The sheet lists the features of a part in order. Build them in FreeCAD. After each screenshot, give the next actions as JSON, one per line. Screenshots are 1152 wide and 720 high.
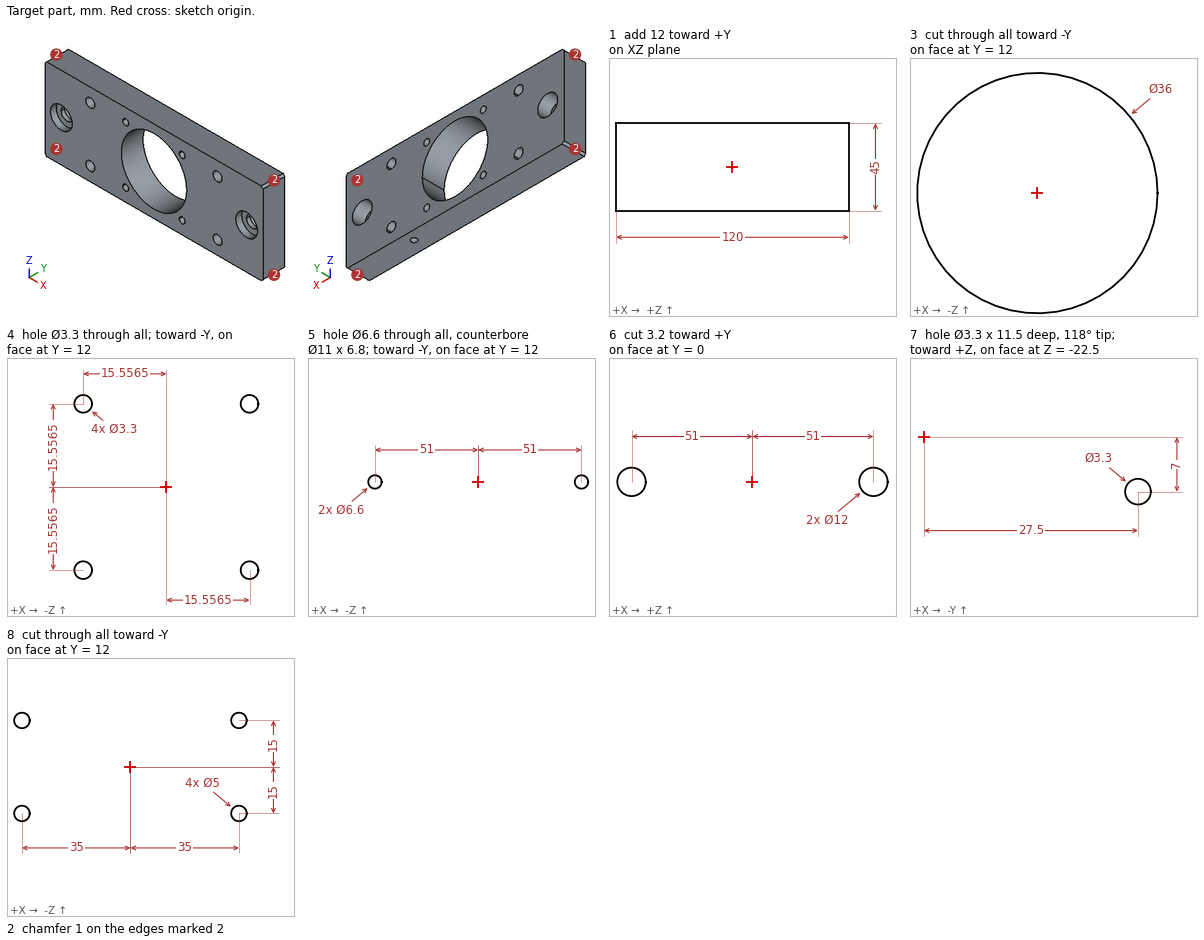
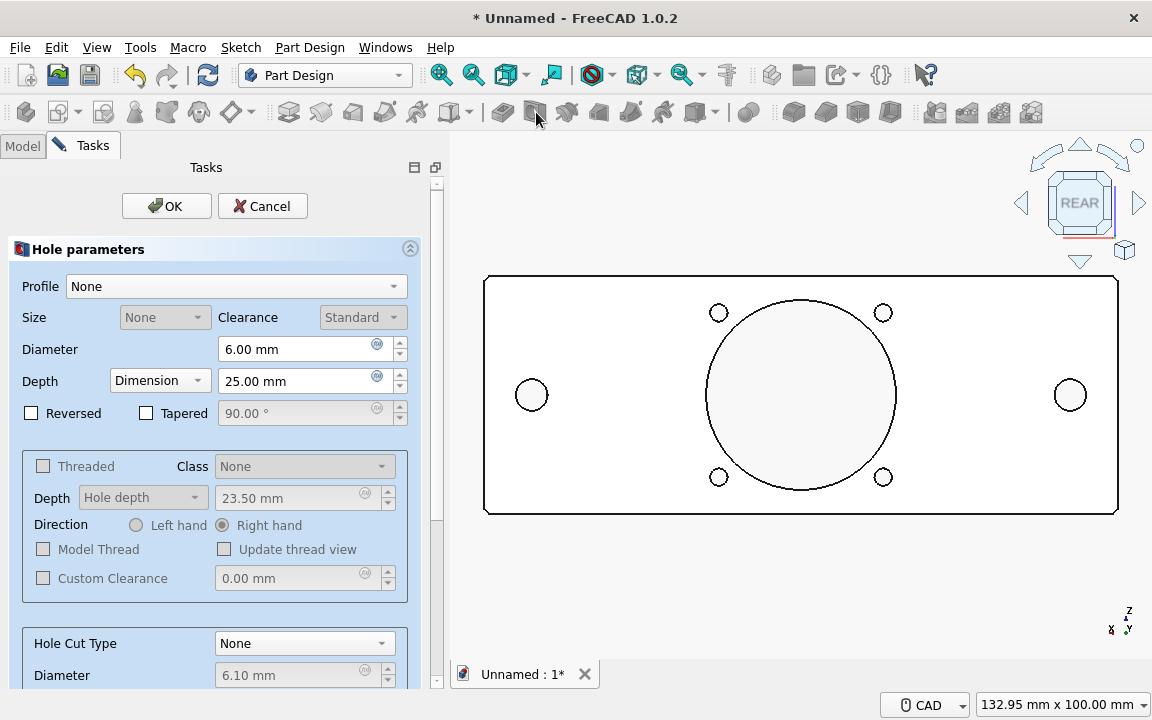
{"action": "triple_click", "coordinate": [305, 349]}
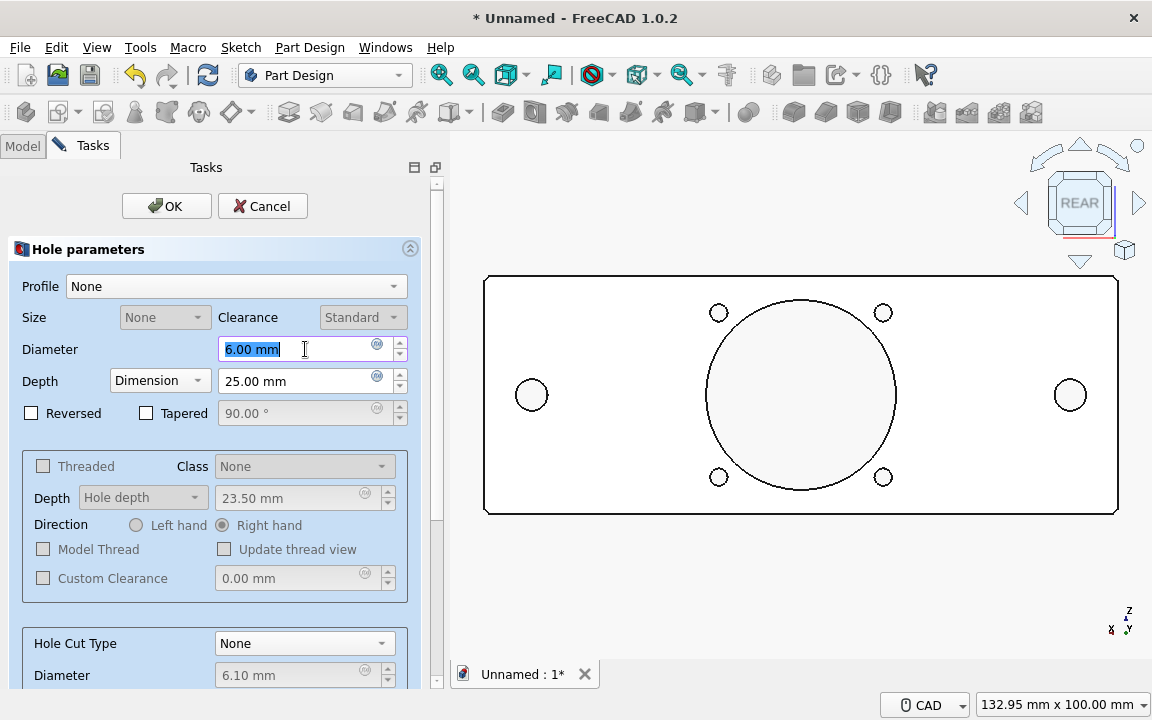
{"action": "type", "text": "6.6"}
{"action": "key", "text": "Tab"}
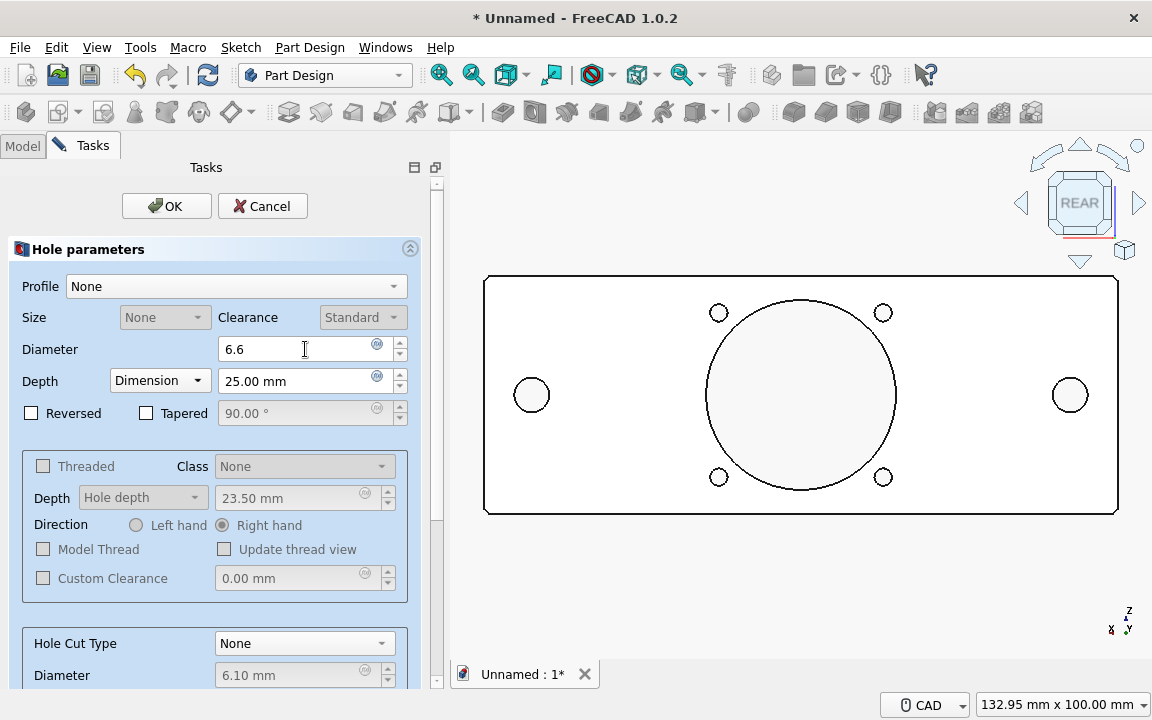
{"action": "left_click", "coordinate": [161, 380]}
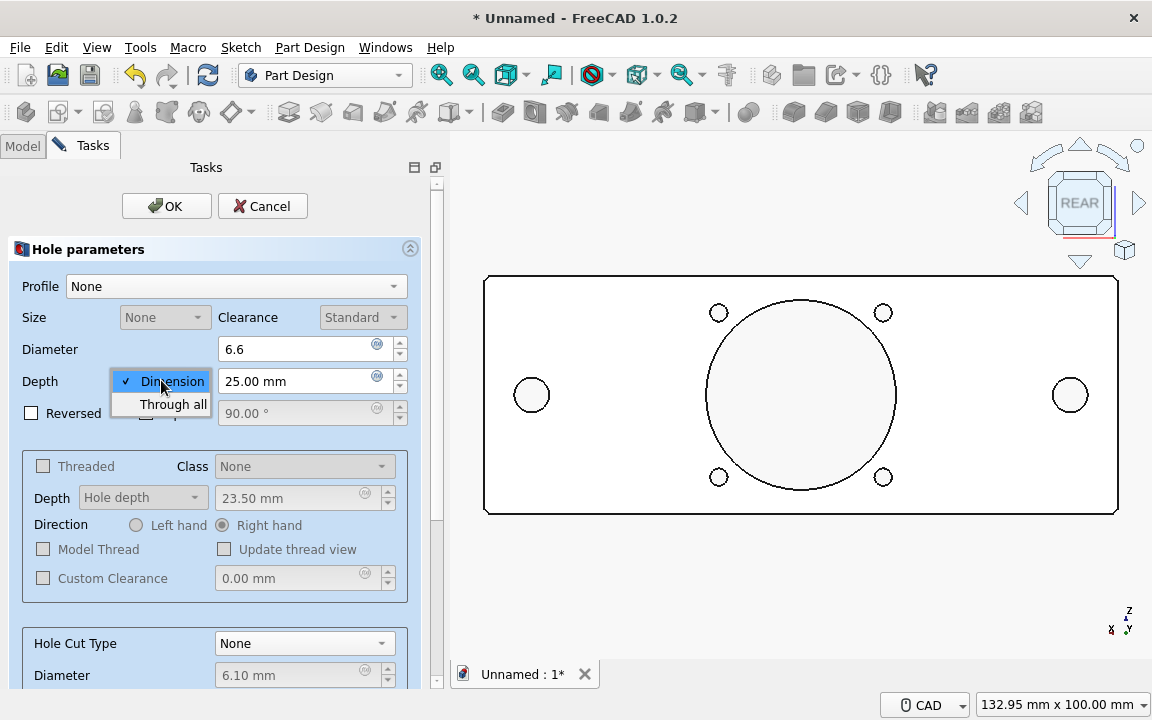
{"action": "left_click", "coordinate": [160, 404]}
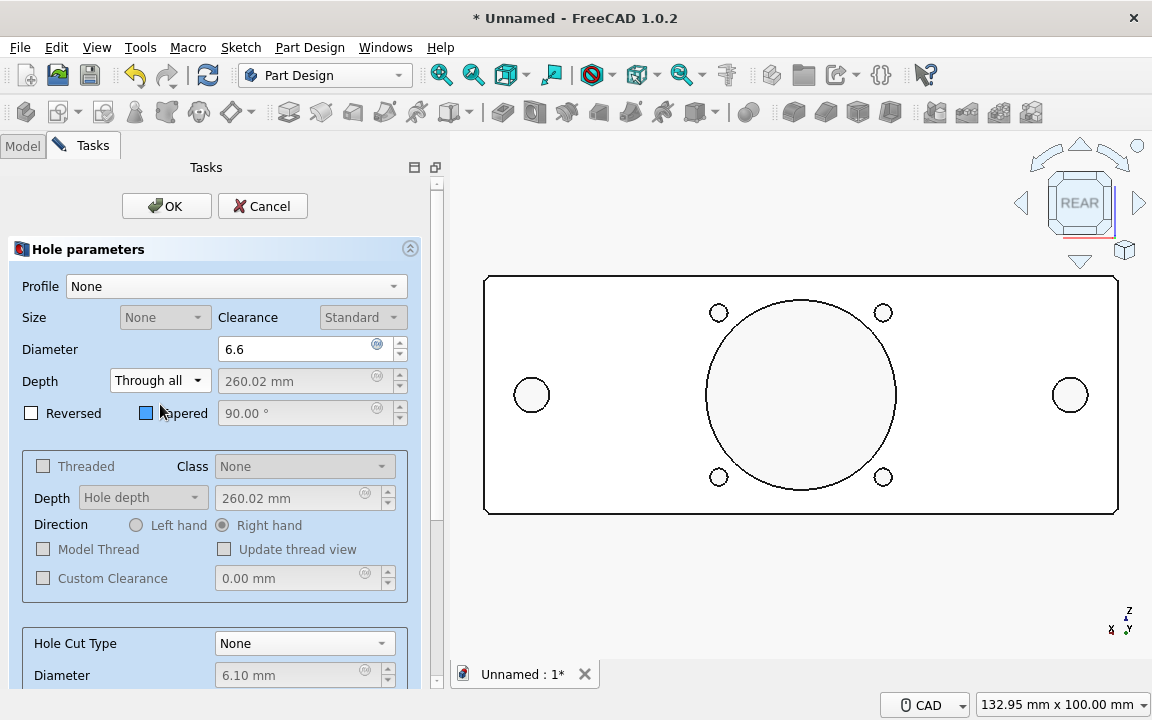
{"action": "left_click", "coordinate": [306, 644]}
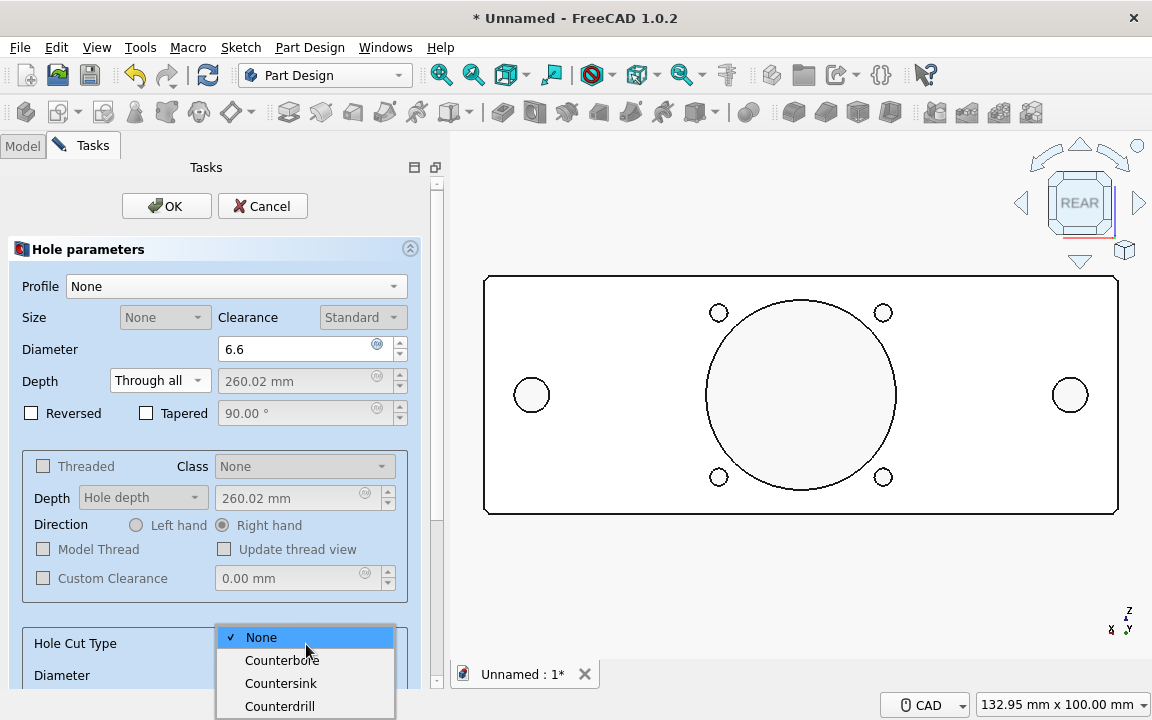
{"action": "left_click", "coordinate": [304, 660]}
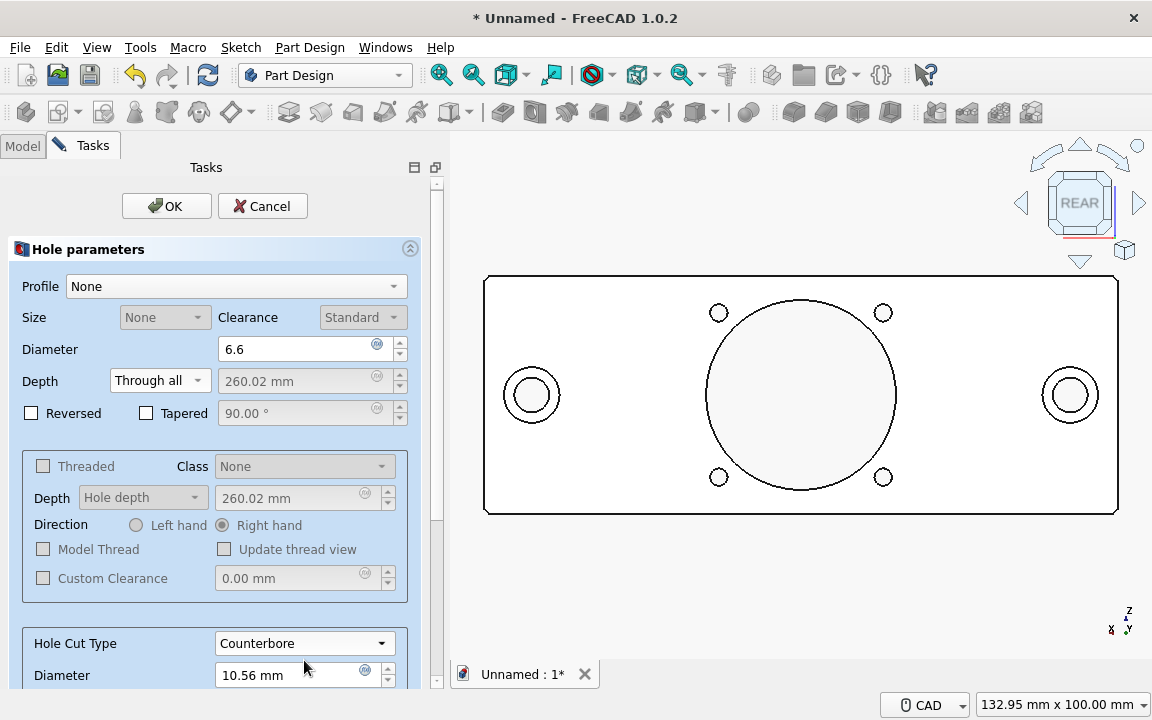
{"action": "triple_click", "coordinate": [298, 675]}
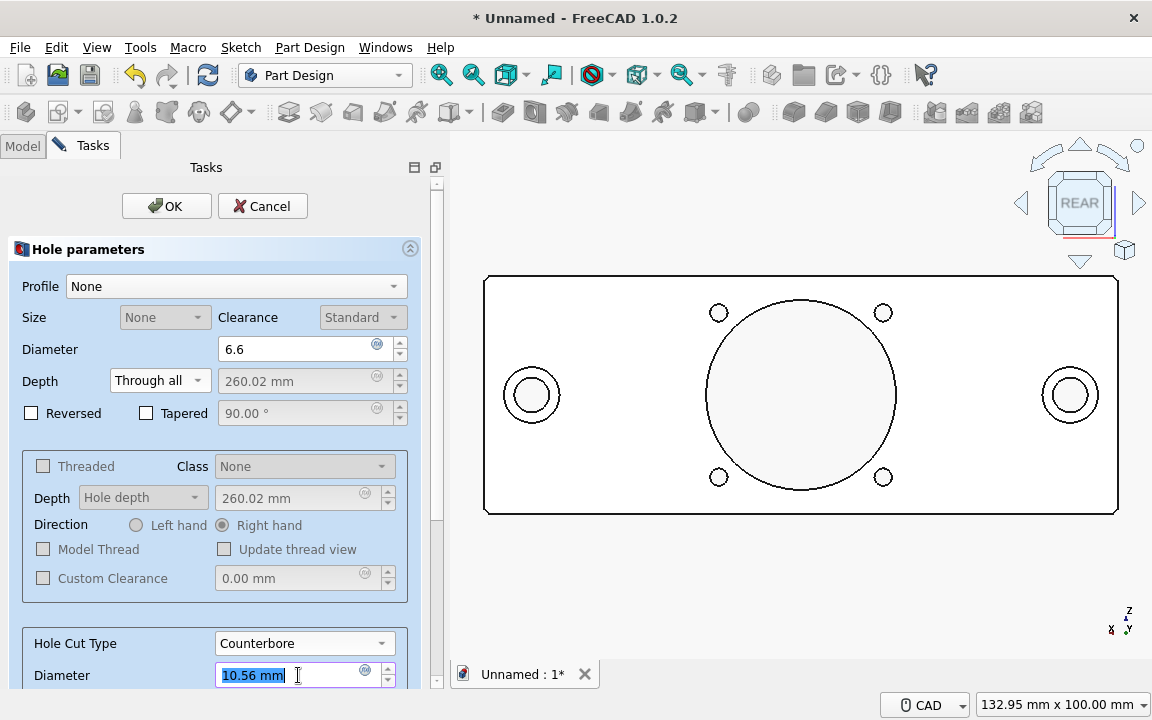
{"action": "type", "text": "11"}
{"action": "key", "text": "Tab"}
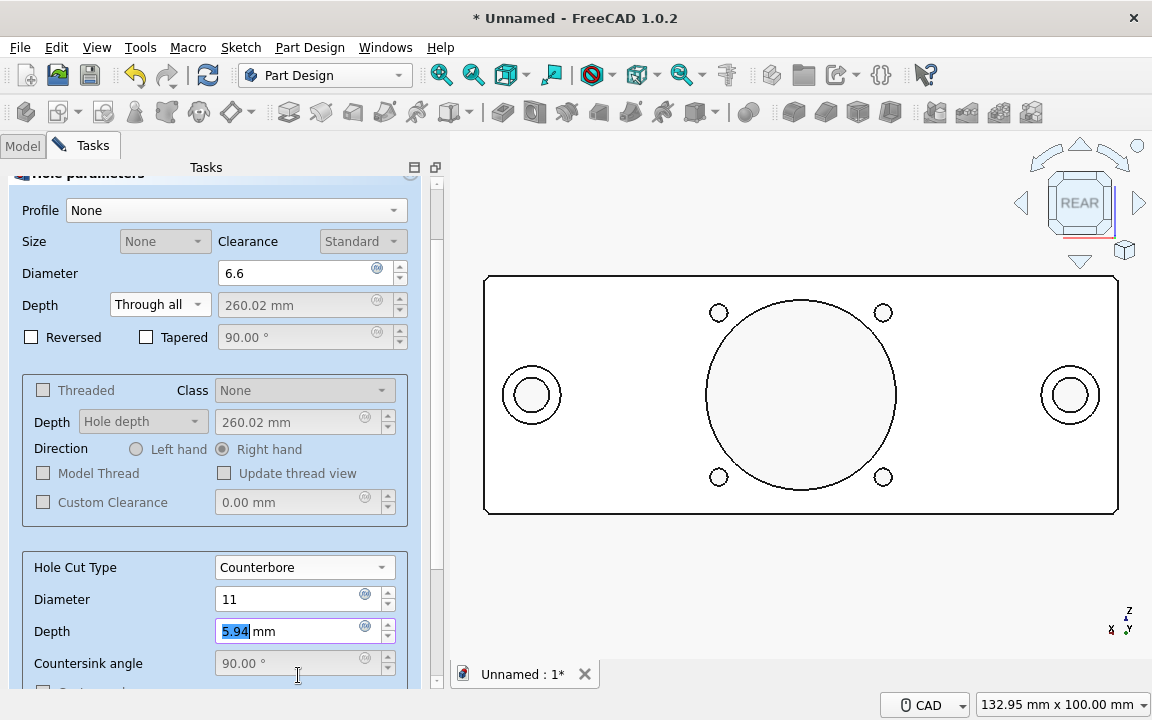
{"action": "type", "text": "6.8"}
{"action": "key", "text": "Tab"}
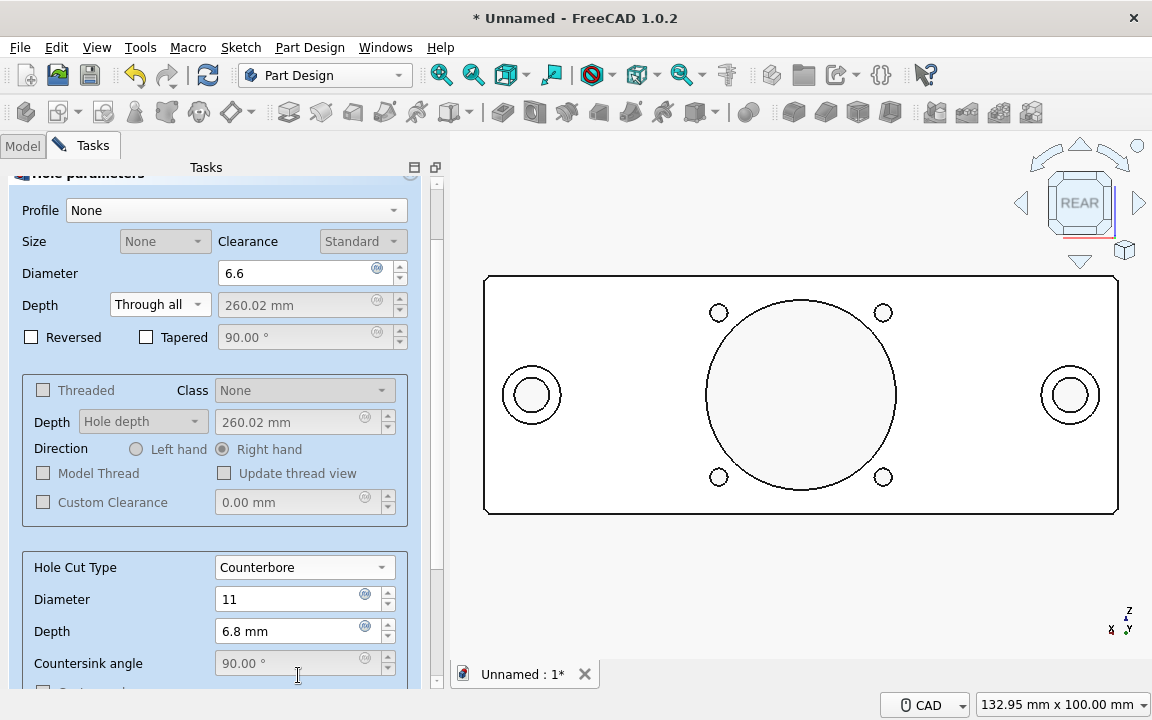
{"action": "scroll", "coordinate": [437, 432], "scroll_direction": "up", "scroll_amount": 3}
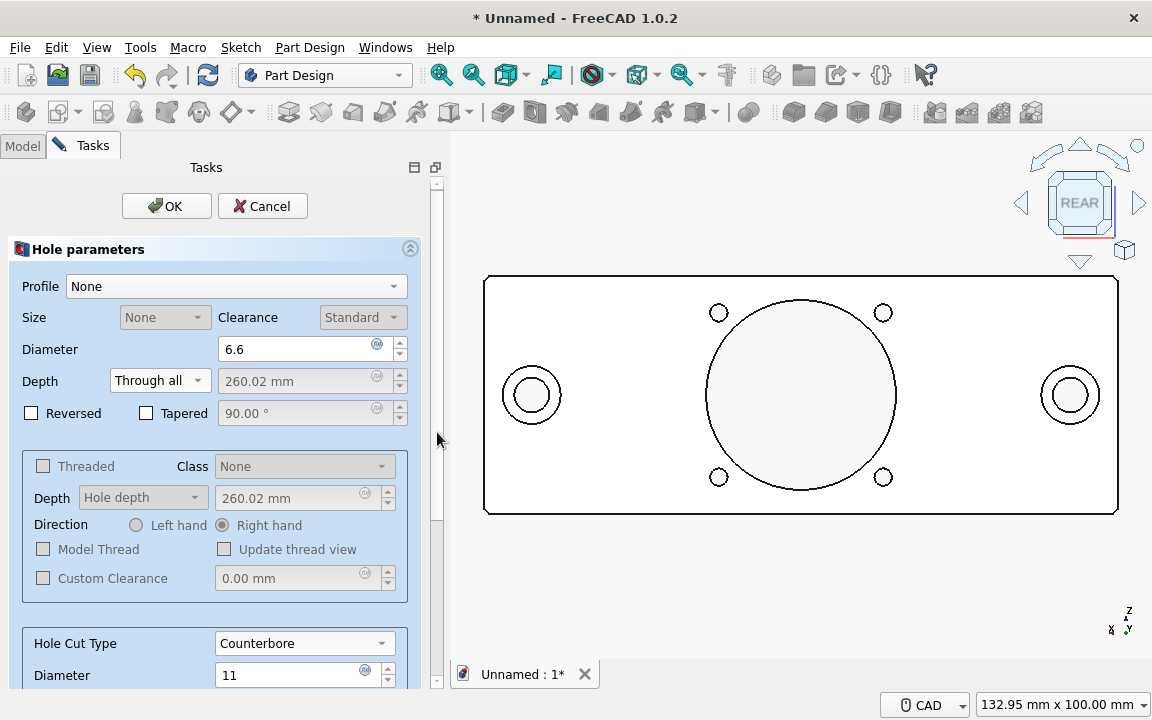
{"action": "left_click", "coordinate": [167, 206]}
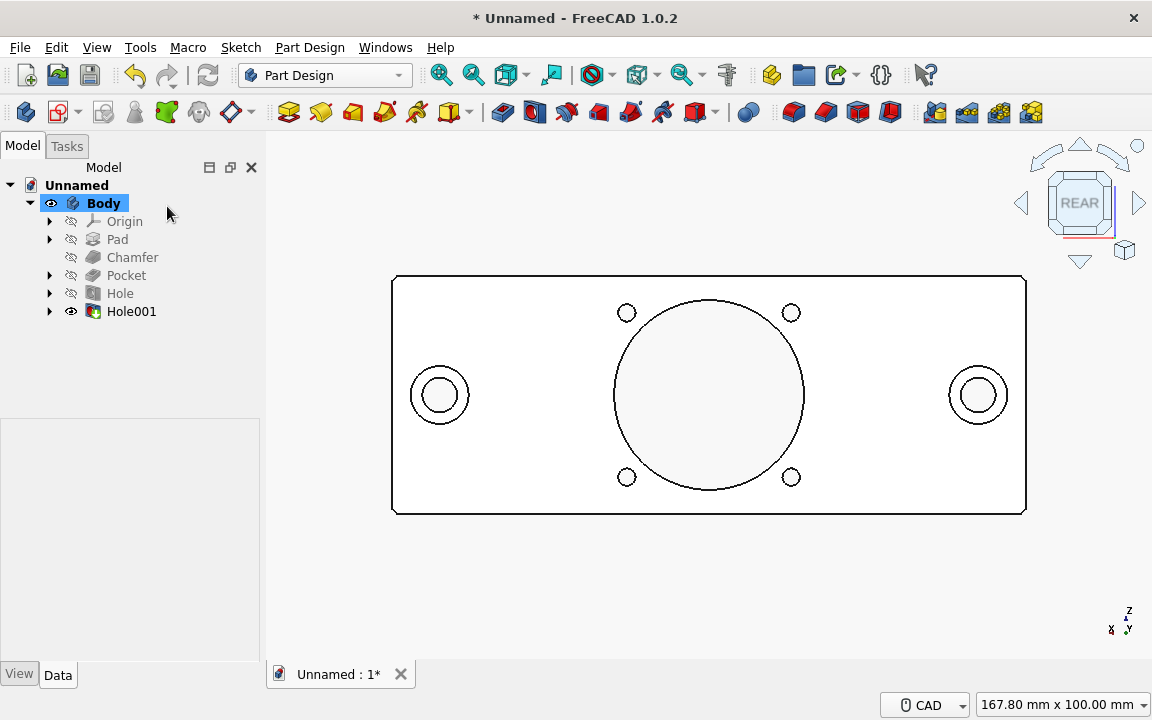
{"action": "key", "text": "0"}